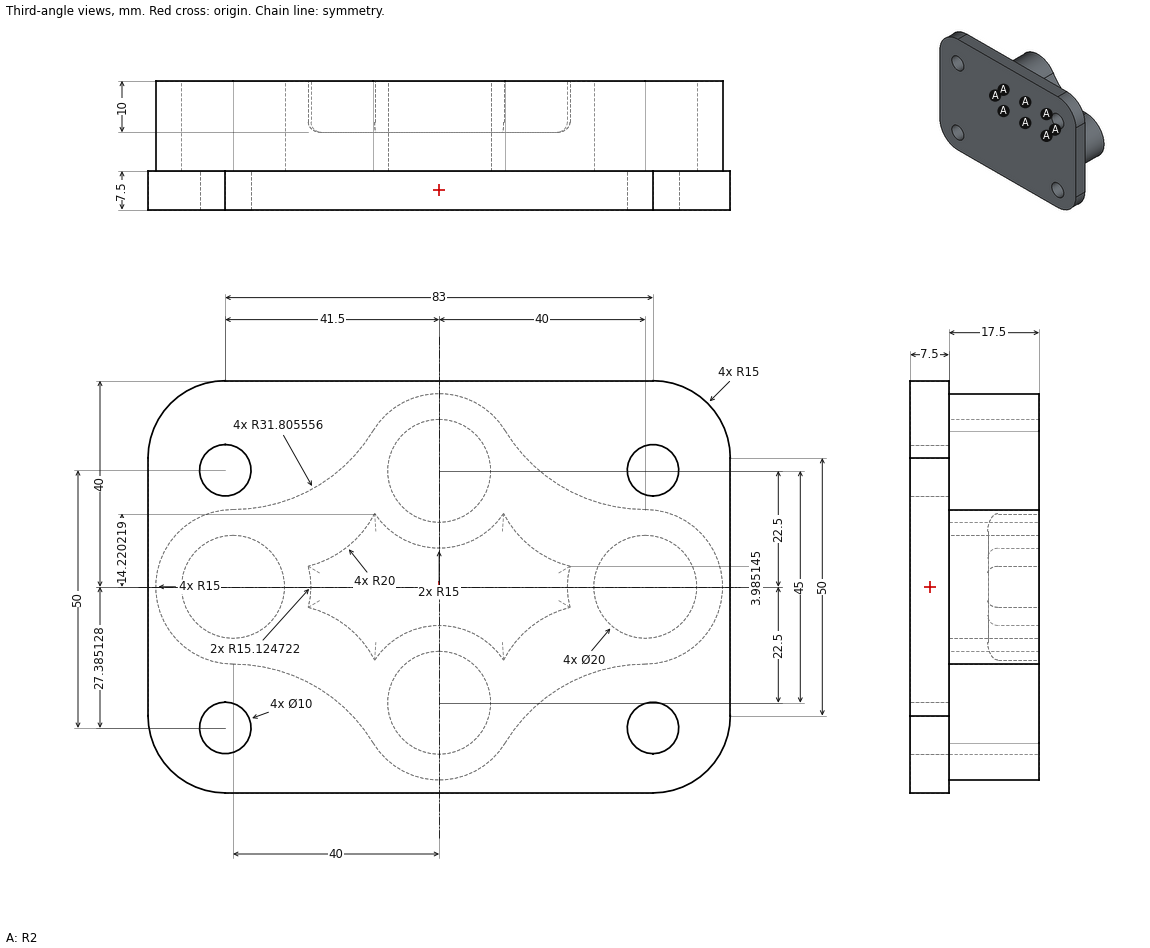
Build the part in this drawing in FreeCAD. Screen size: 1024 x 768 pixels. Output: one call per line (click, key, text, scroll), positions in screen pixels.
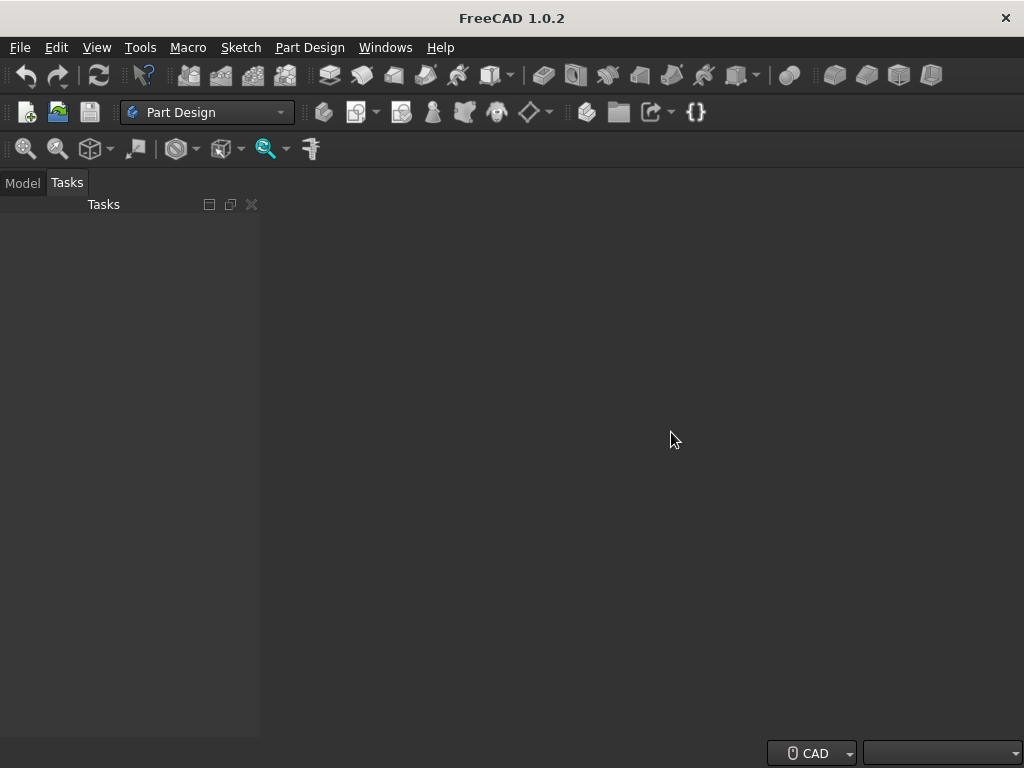
click(26, 112)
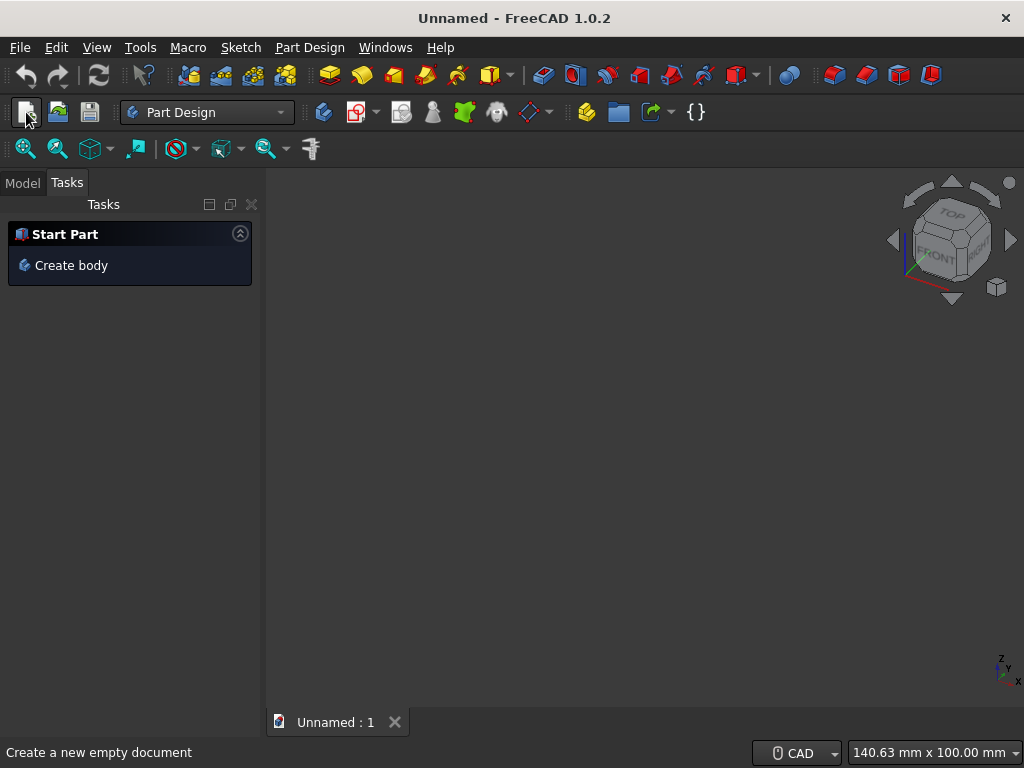
click(356, 112)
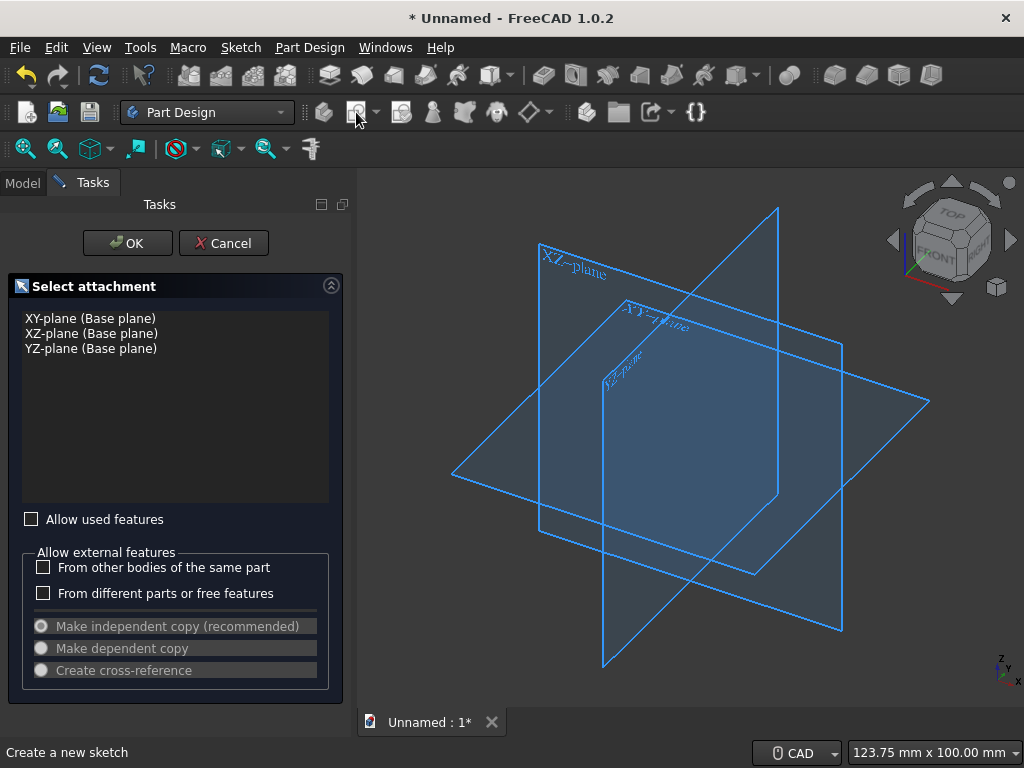
click(82, 334)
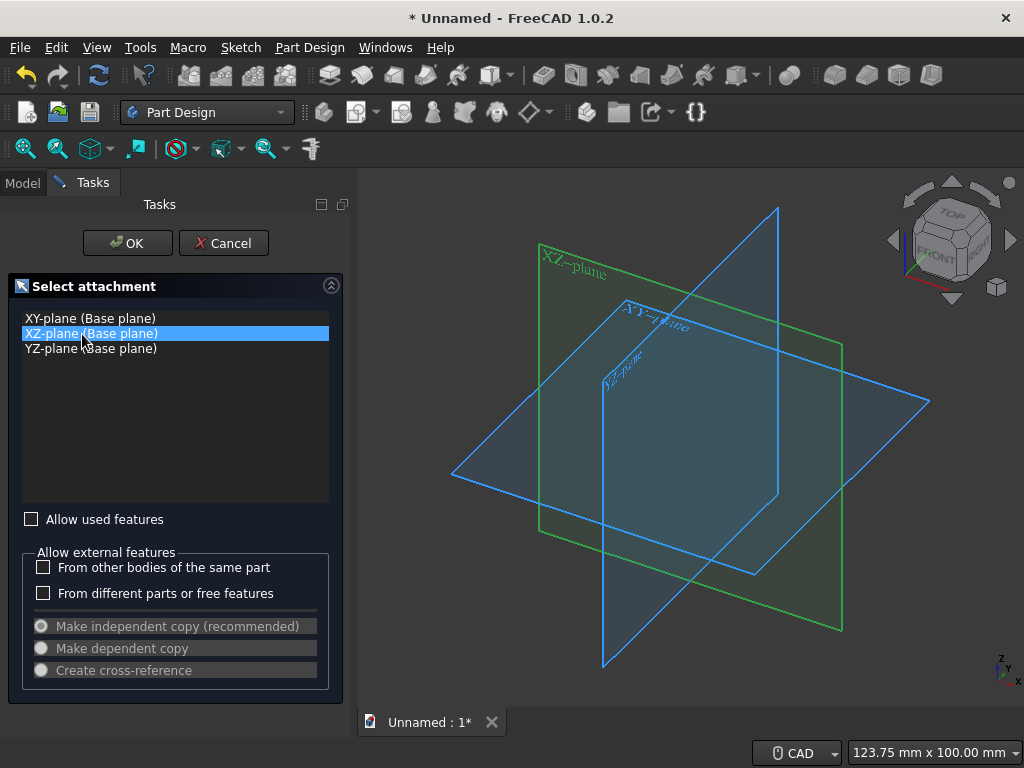
click(128, 243)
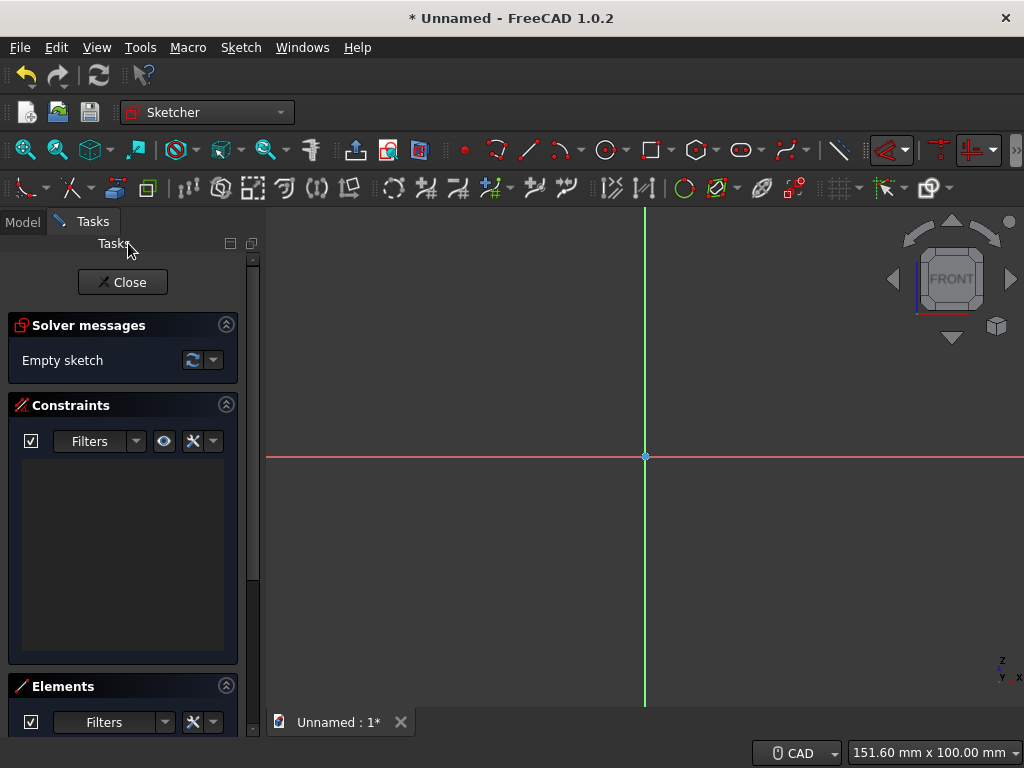
scroll(437, 457, down, 2)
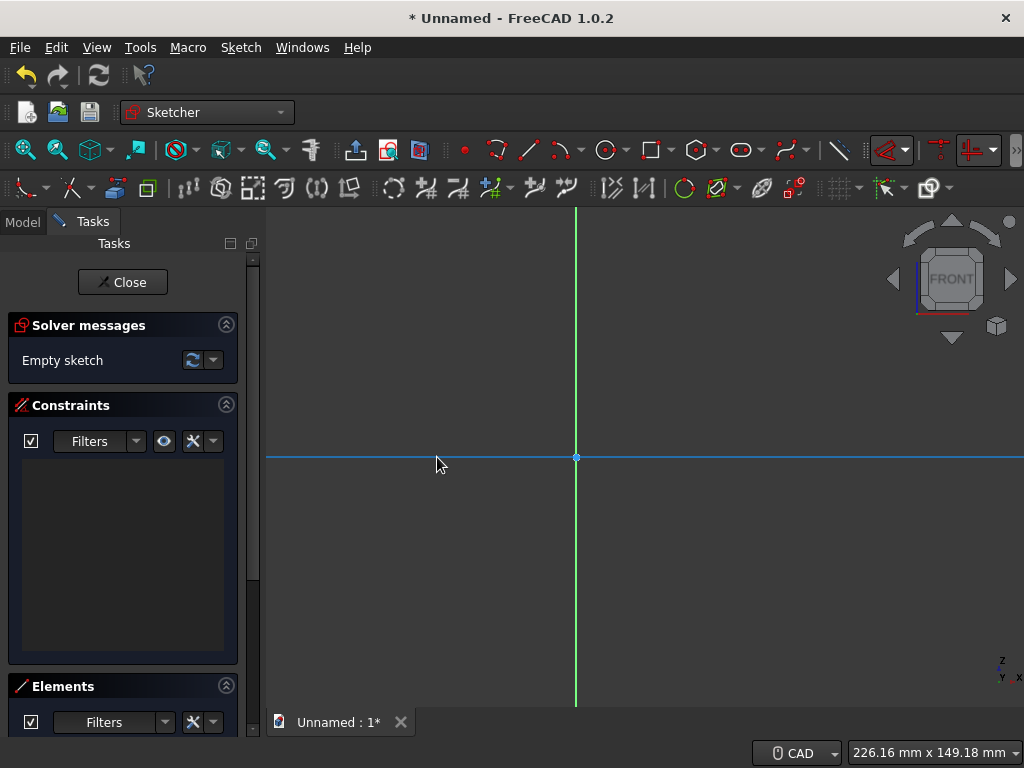
click(530, 150)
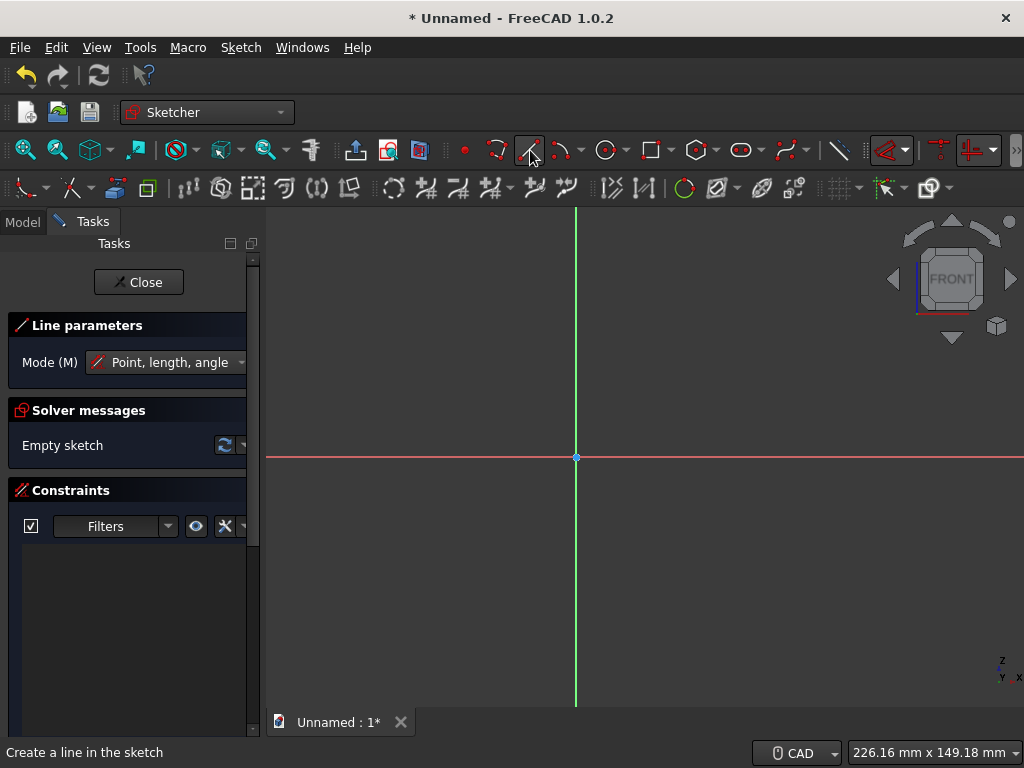
click(437, 323)
click(716, 323)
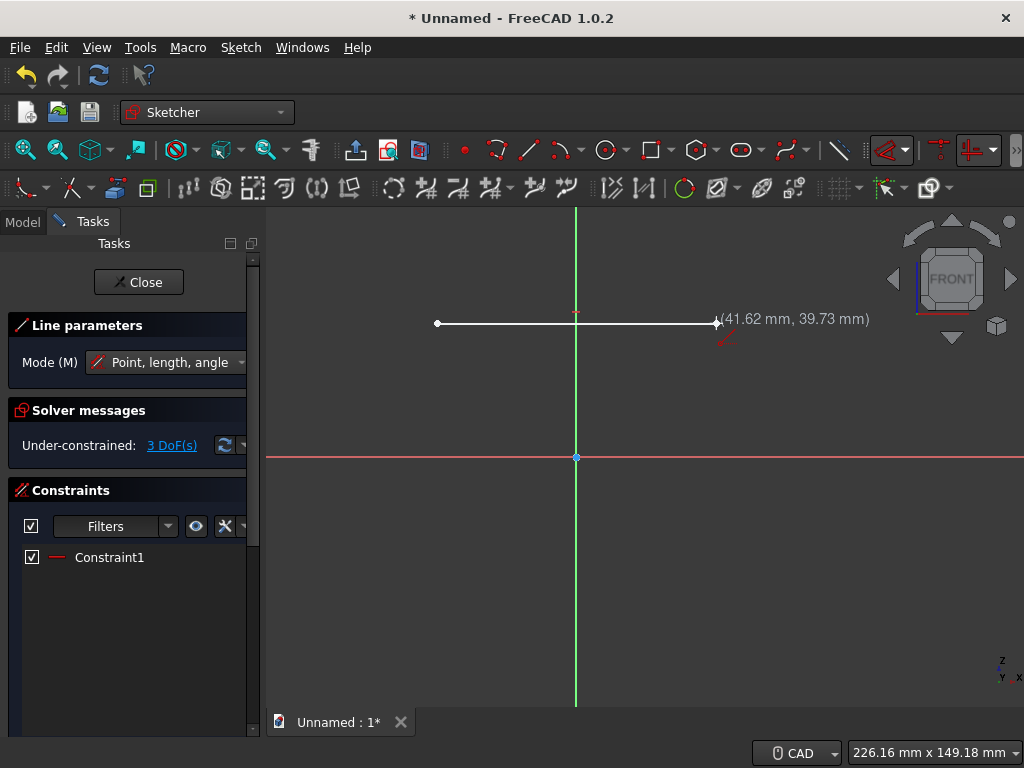
click(766, 373)
click(766, 541)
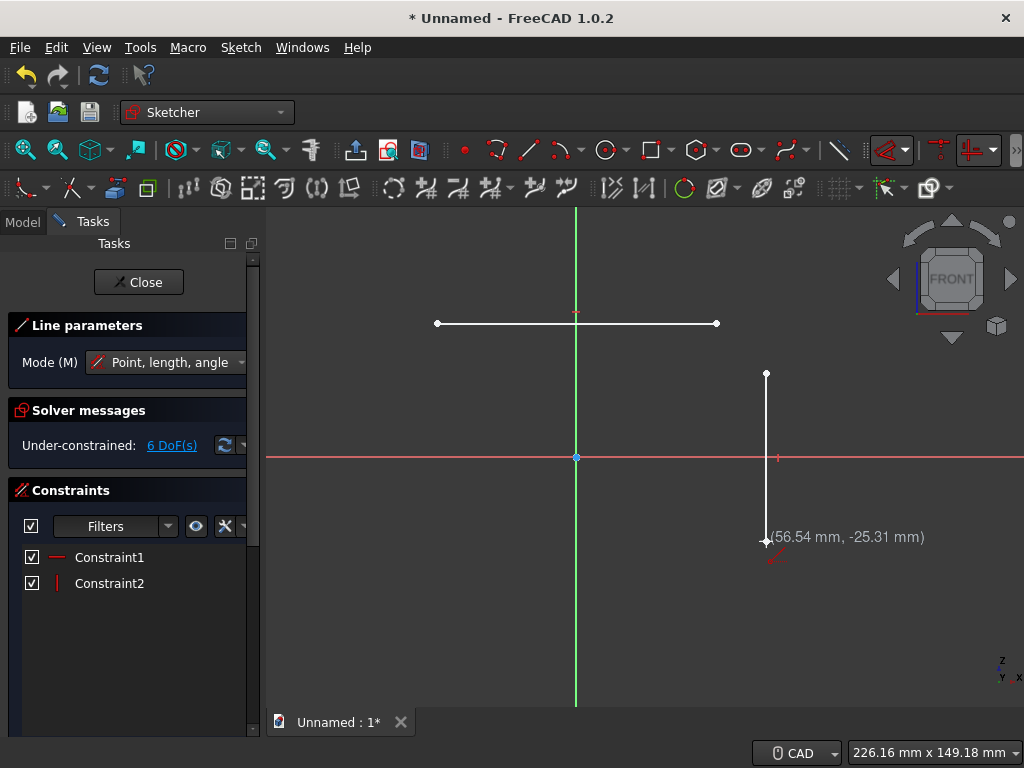
click(716, 591)
click(437, 591)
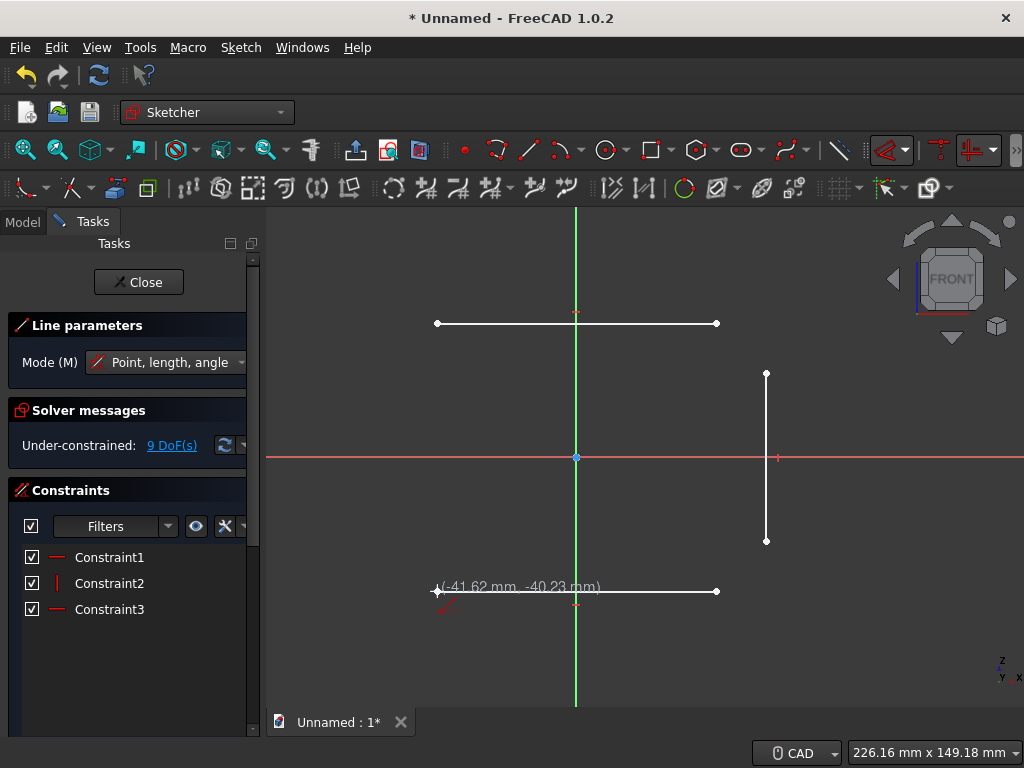
click(387, 541)
click(387, 373)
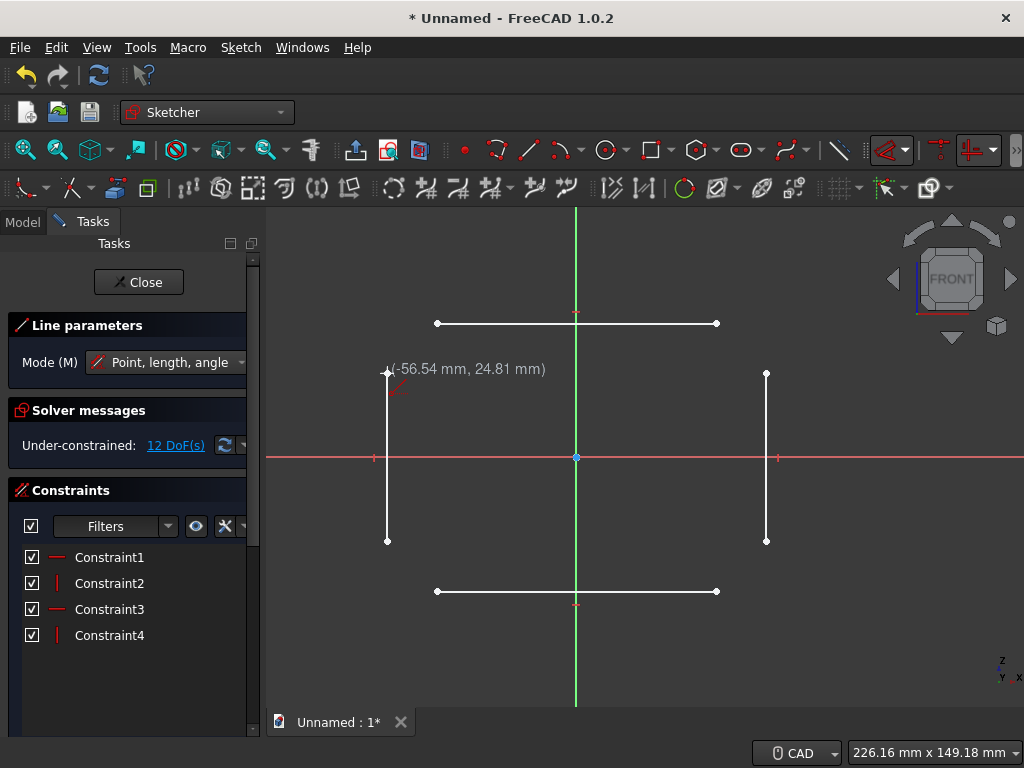
click(584, 150)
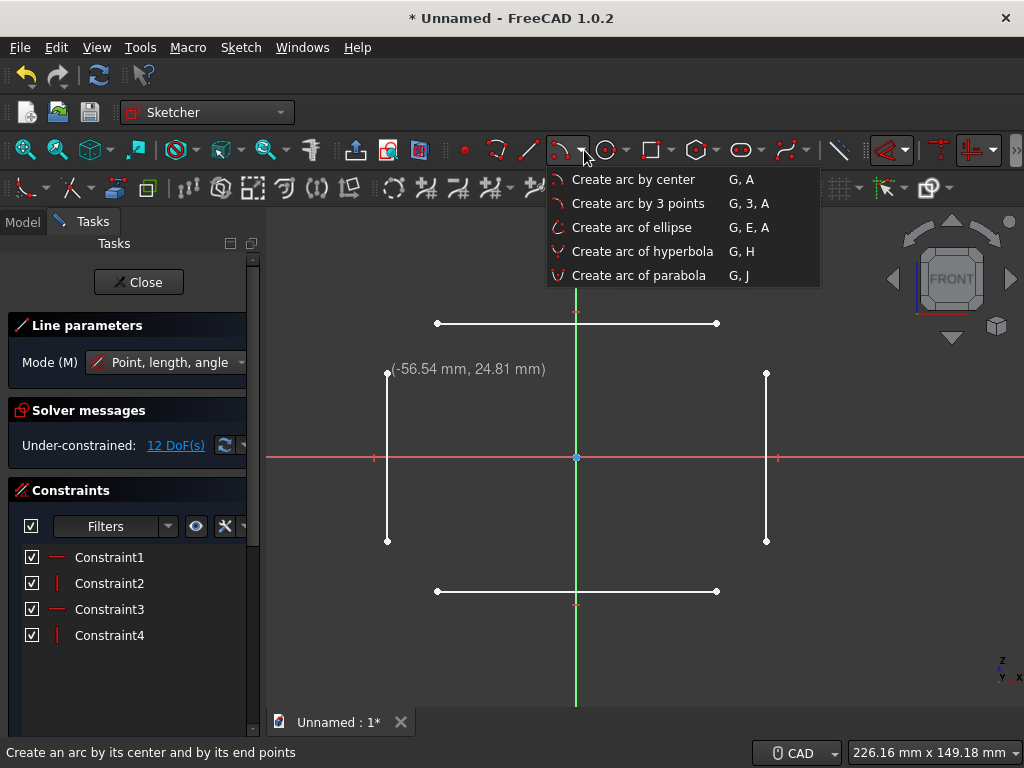
click(684, 203)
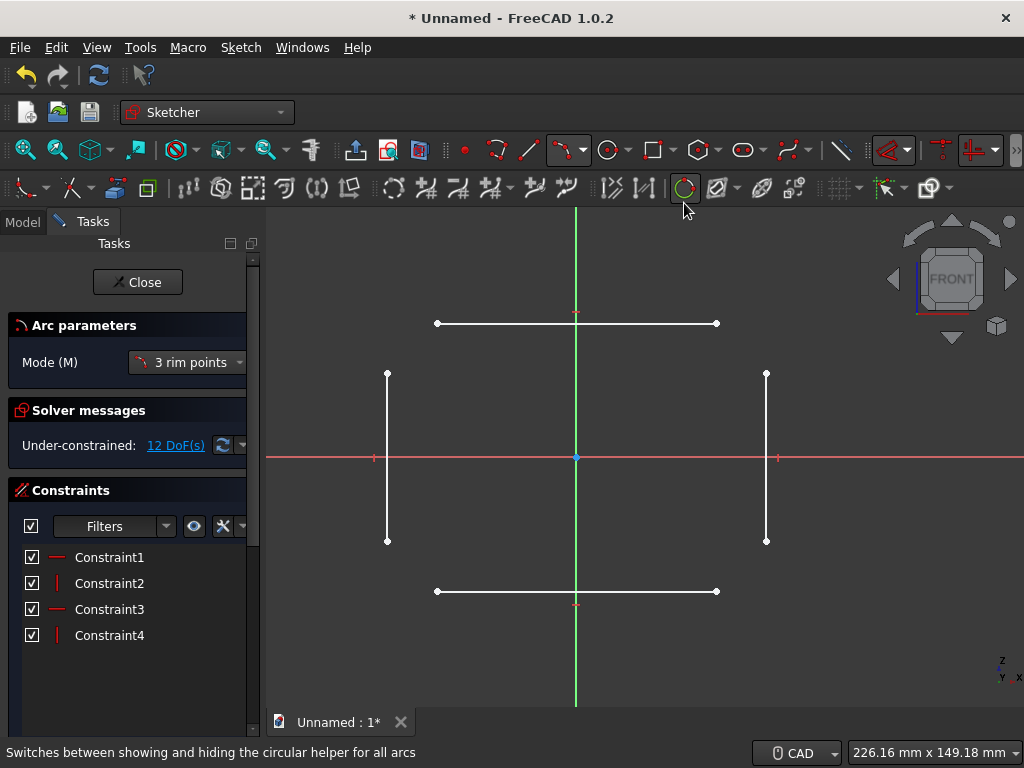
click(716, 324)
click(766, 374)
click(751, 338)